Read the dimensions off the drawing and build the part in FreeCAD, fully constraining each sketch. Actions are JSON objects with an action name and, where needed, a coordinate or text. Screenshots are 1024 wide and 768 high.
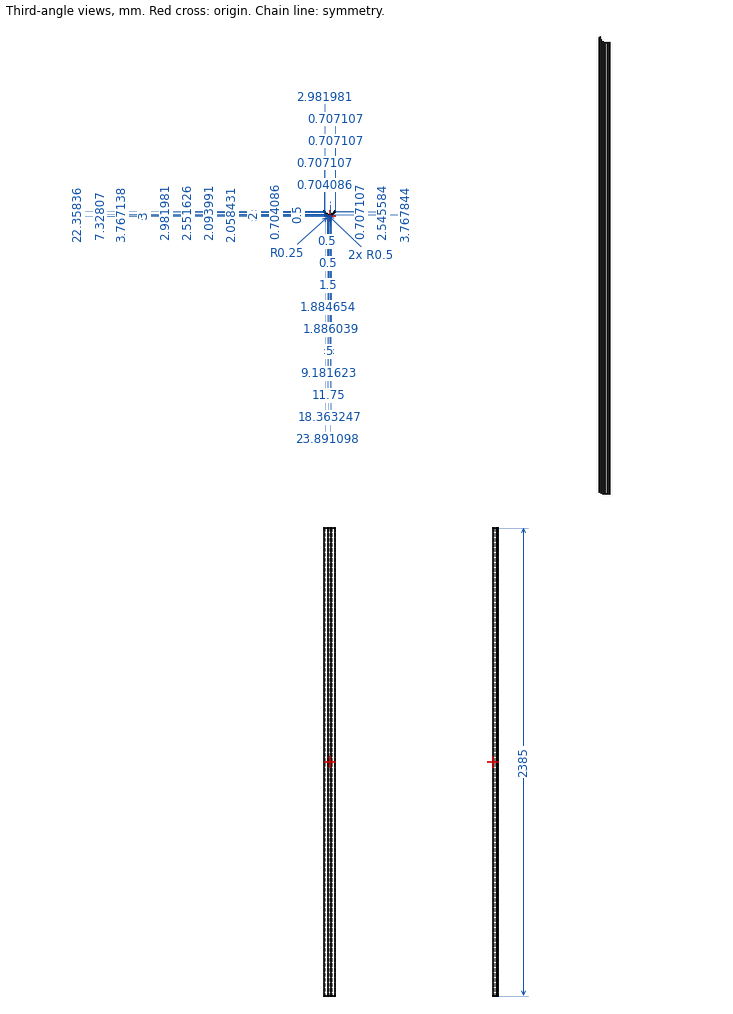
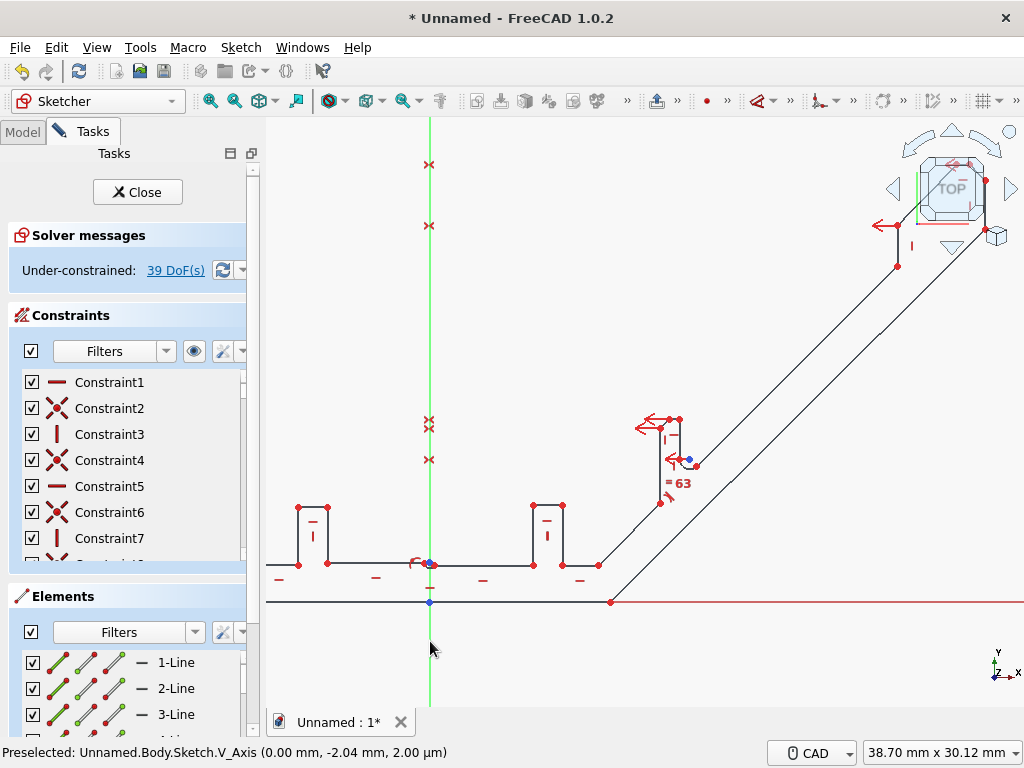
{"action": "left_click", "coordinate": [298, 565]}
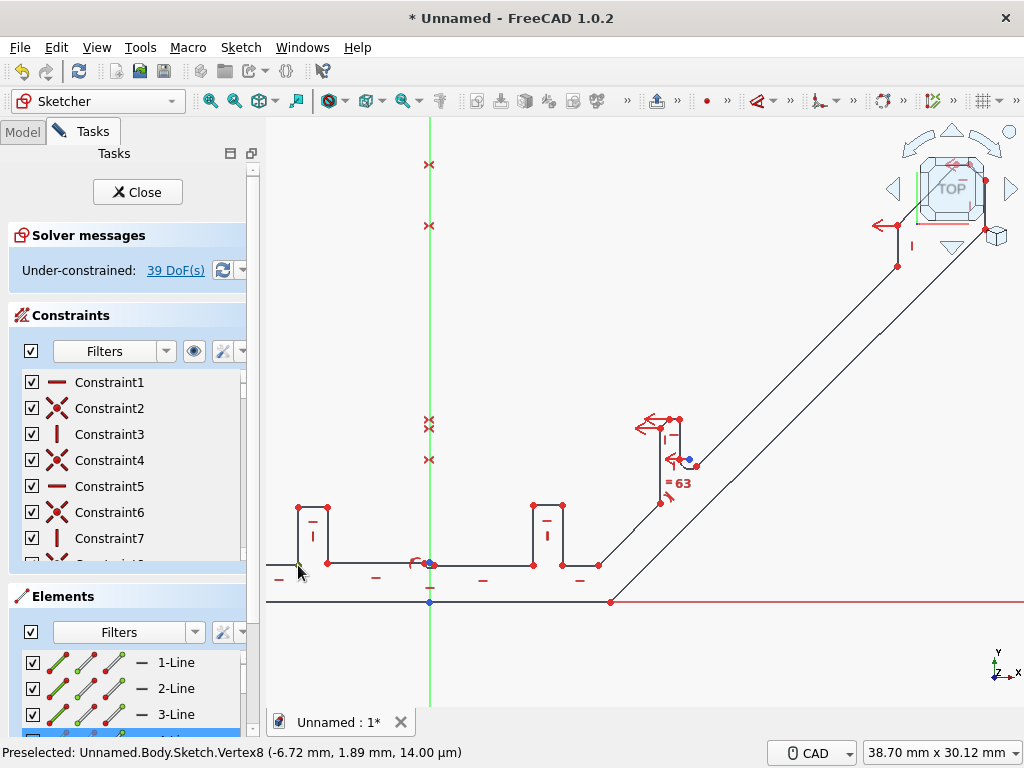
{"action": "left_click", "coordinate": [563, 566]}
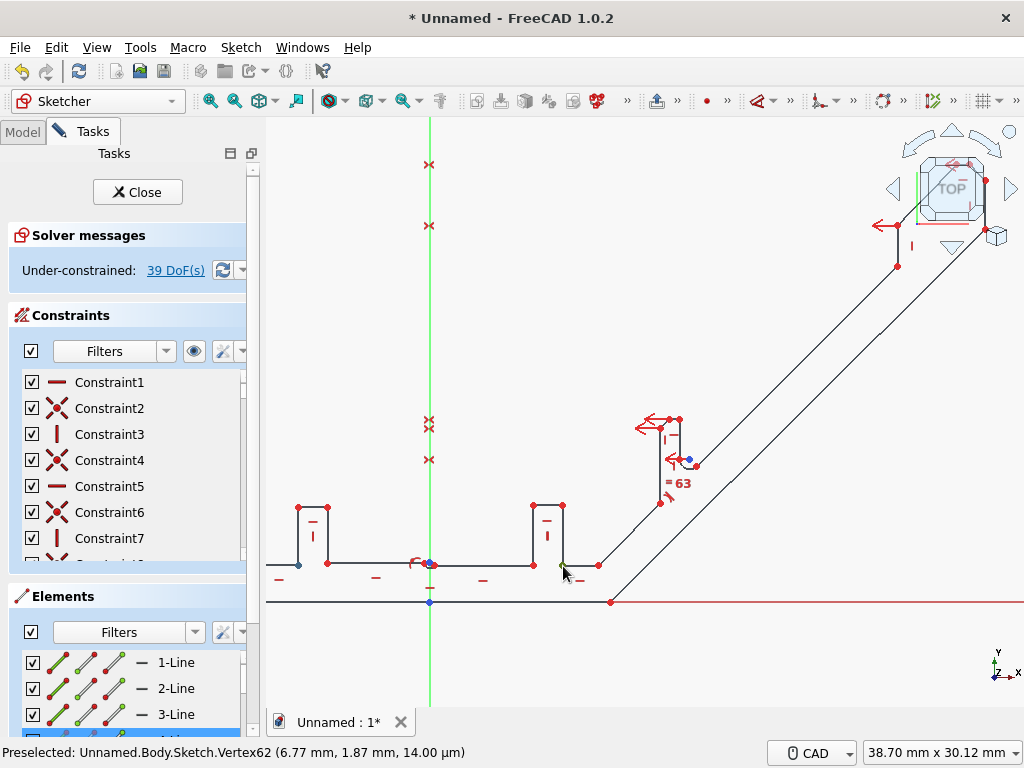
{"action": "left_click", "coordinate": [430, 641]}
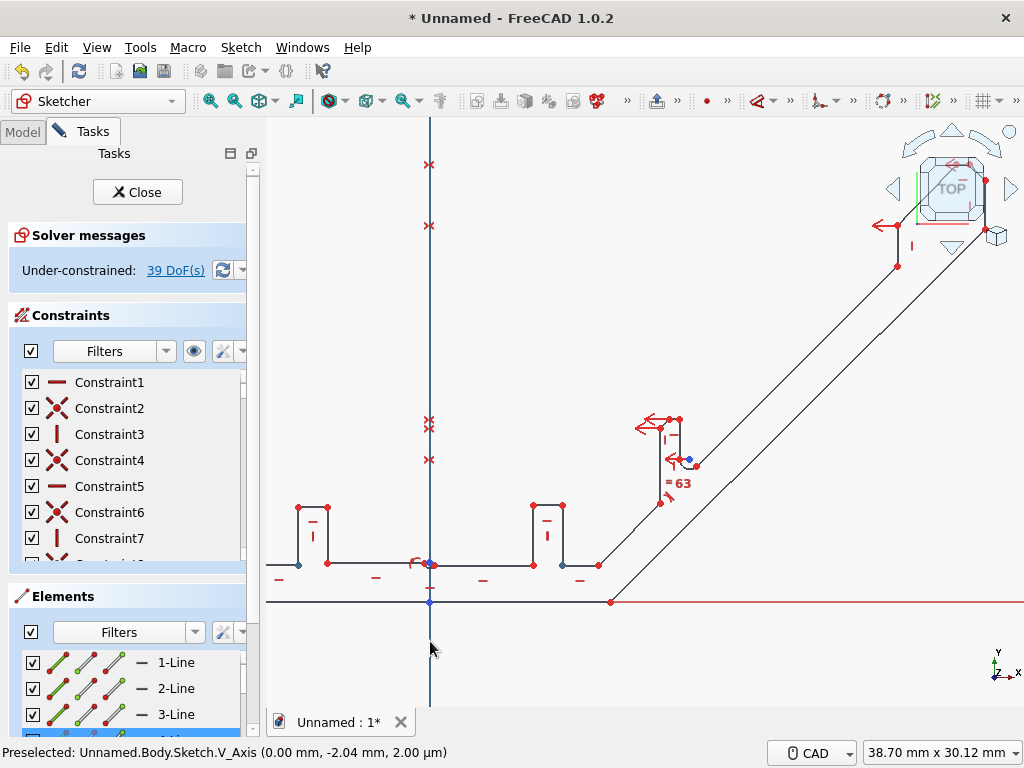
{"action": "key", "text": "s"}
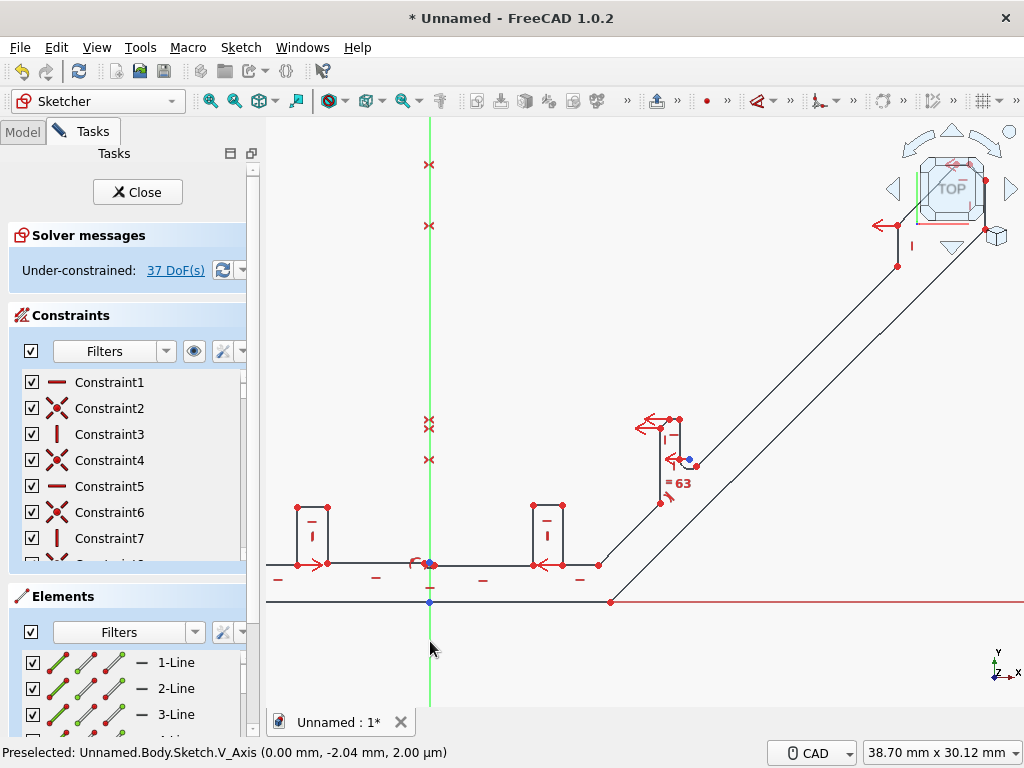
{"action": "left_click", "coordinate": [328, 507]}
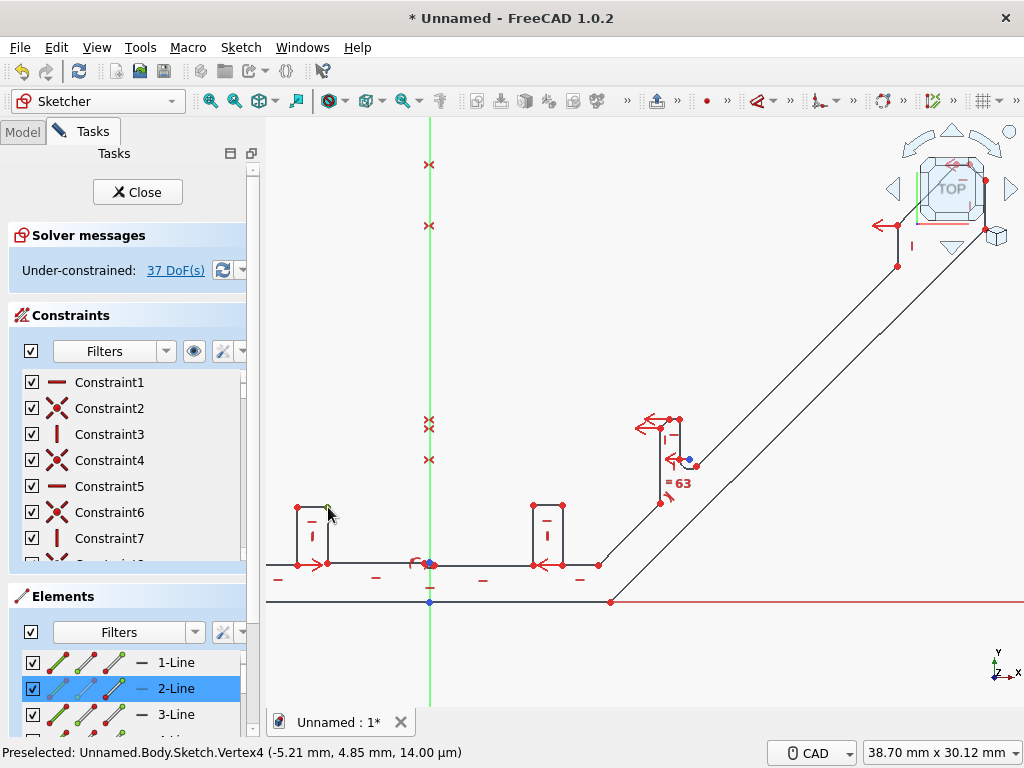
{"action": "left_click", "coordinate": [533, 505]}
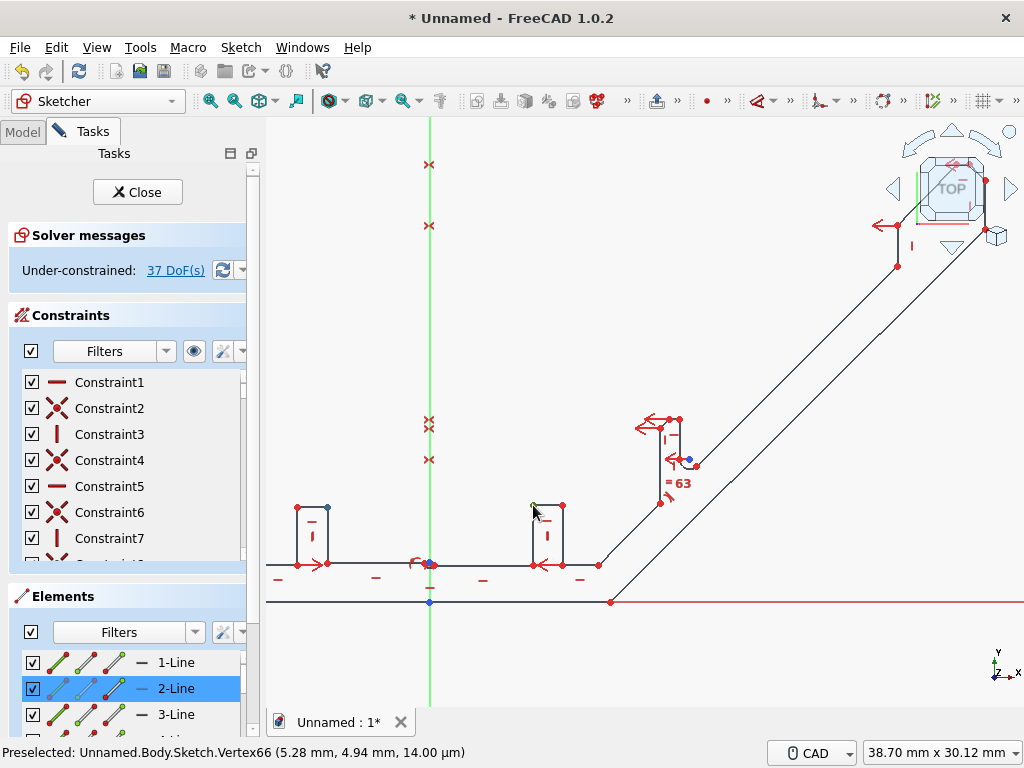
{"action": "left_click", "coordinate": [430, 641]}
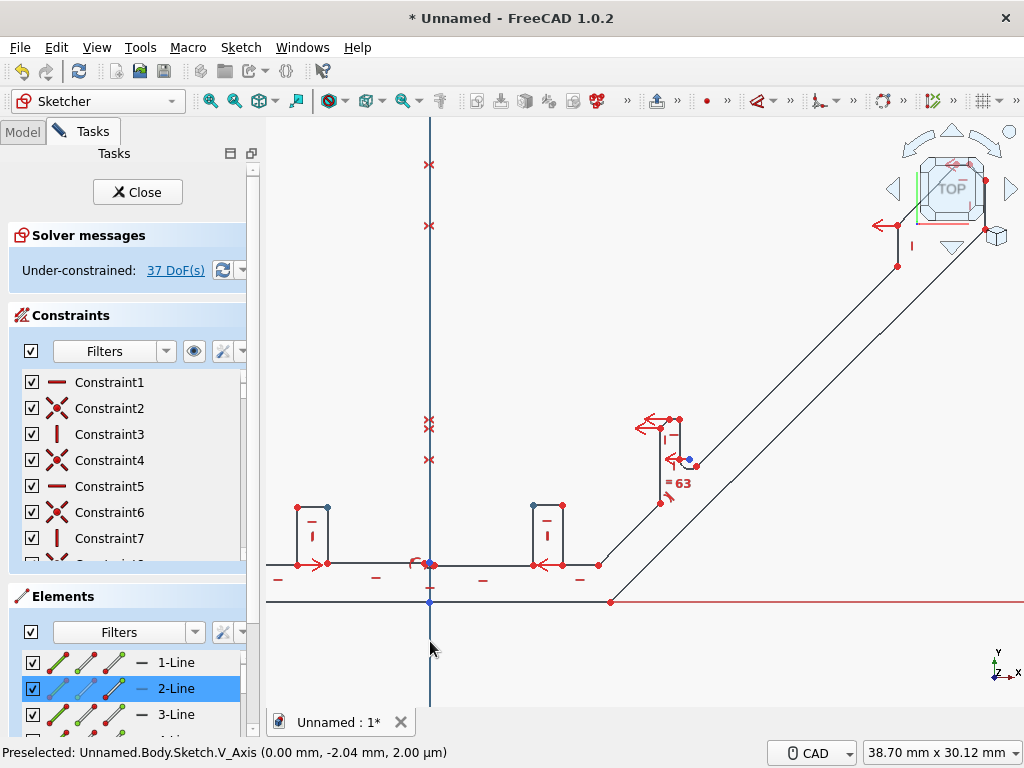
{"action": "key", "text": "s"}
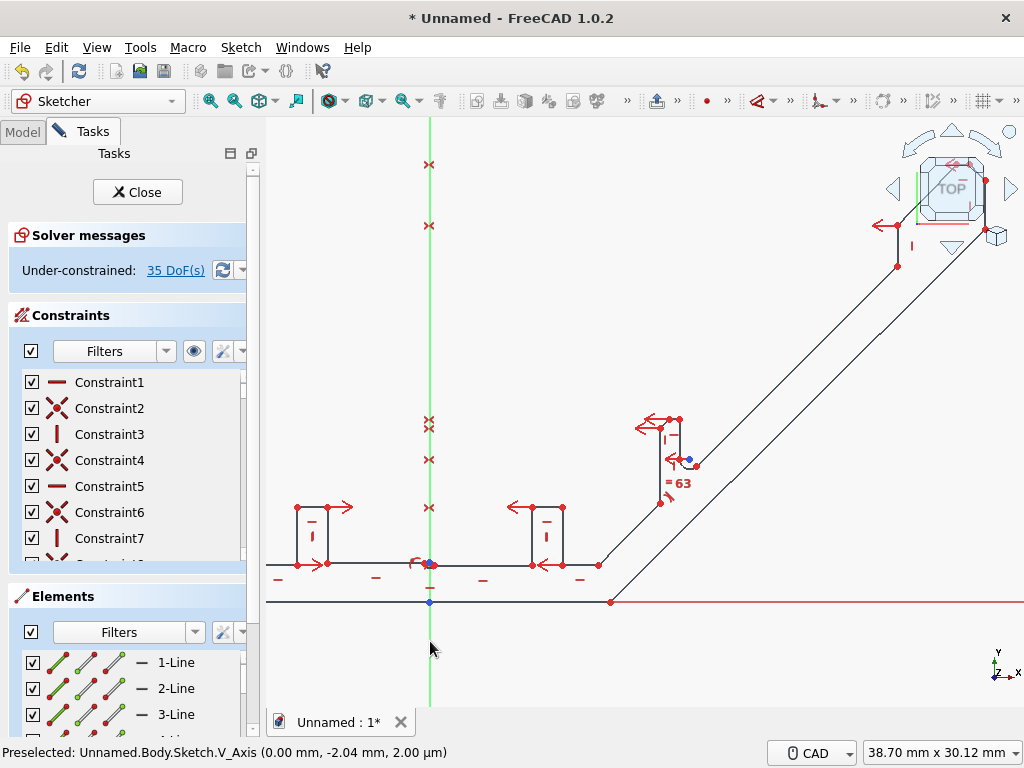
{"action": "key", "text": "d"}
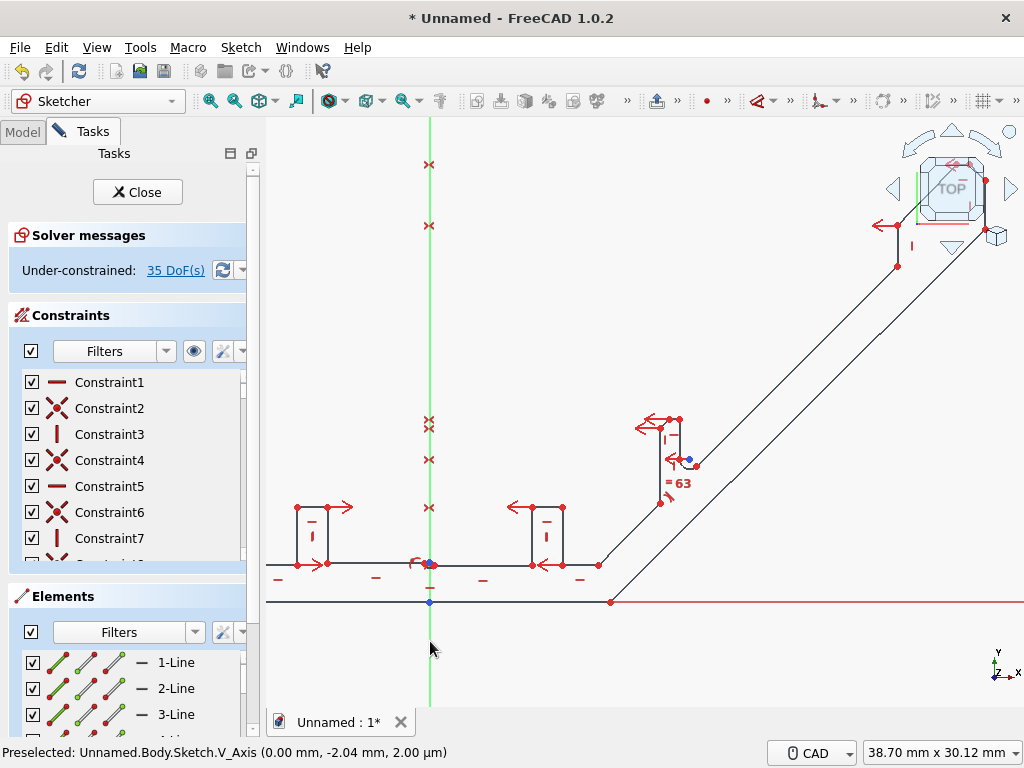
{"action": "scroll", "coordinate": [662, 429], "scroll_direction": "down", "scroll_amount": 5}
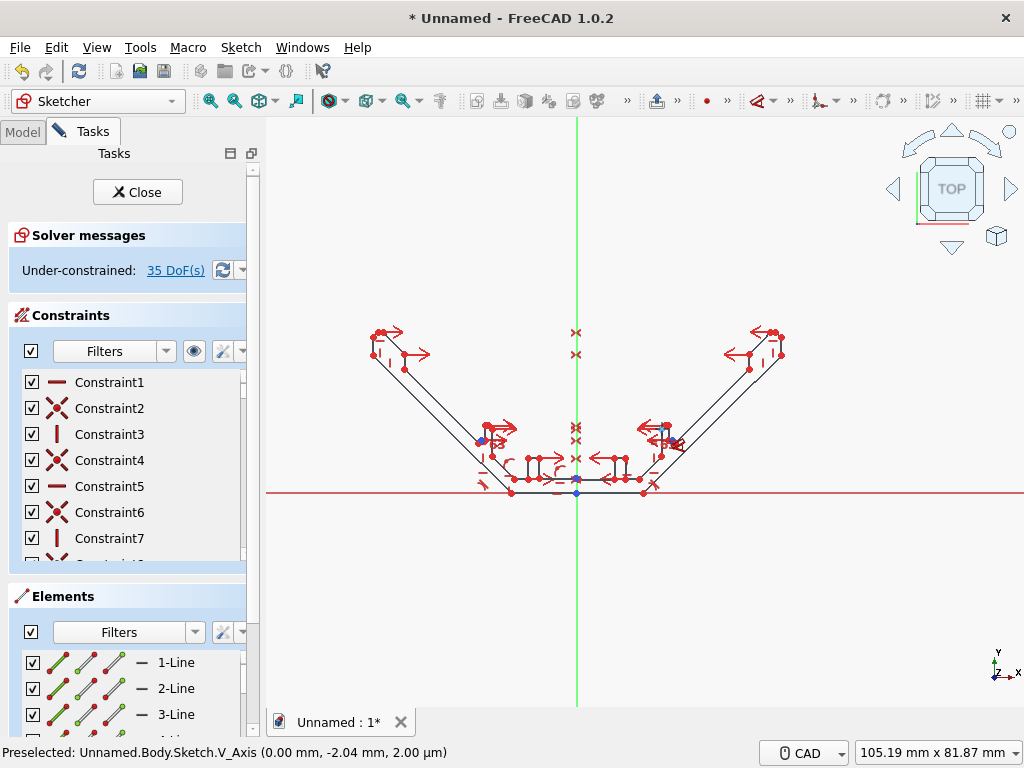
{"action": "scroll", "coordinate": [483, 444], "scroll_direction": "up", "scroll_amount": 12}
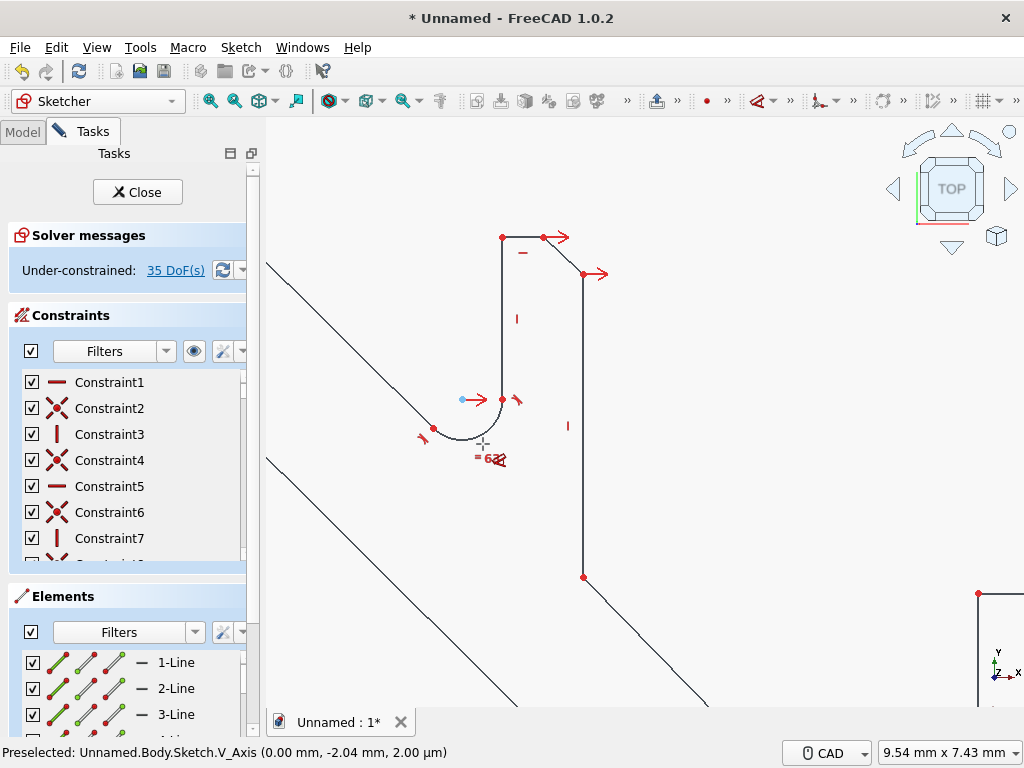
{"action": "left_click", "coordinate": [478, 437]}
{"action": "left_click", "coordinate": [491, 466]}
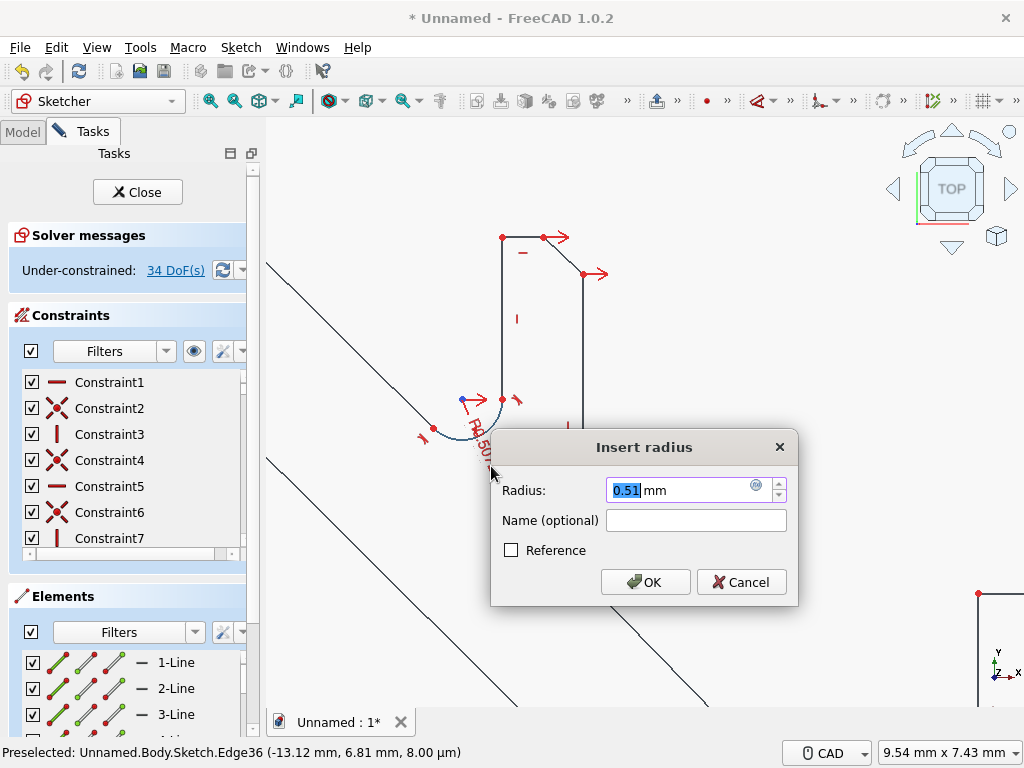
{"action": "type", "text": "0.5"}
{"action": "key", "text": "Return"}